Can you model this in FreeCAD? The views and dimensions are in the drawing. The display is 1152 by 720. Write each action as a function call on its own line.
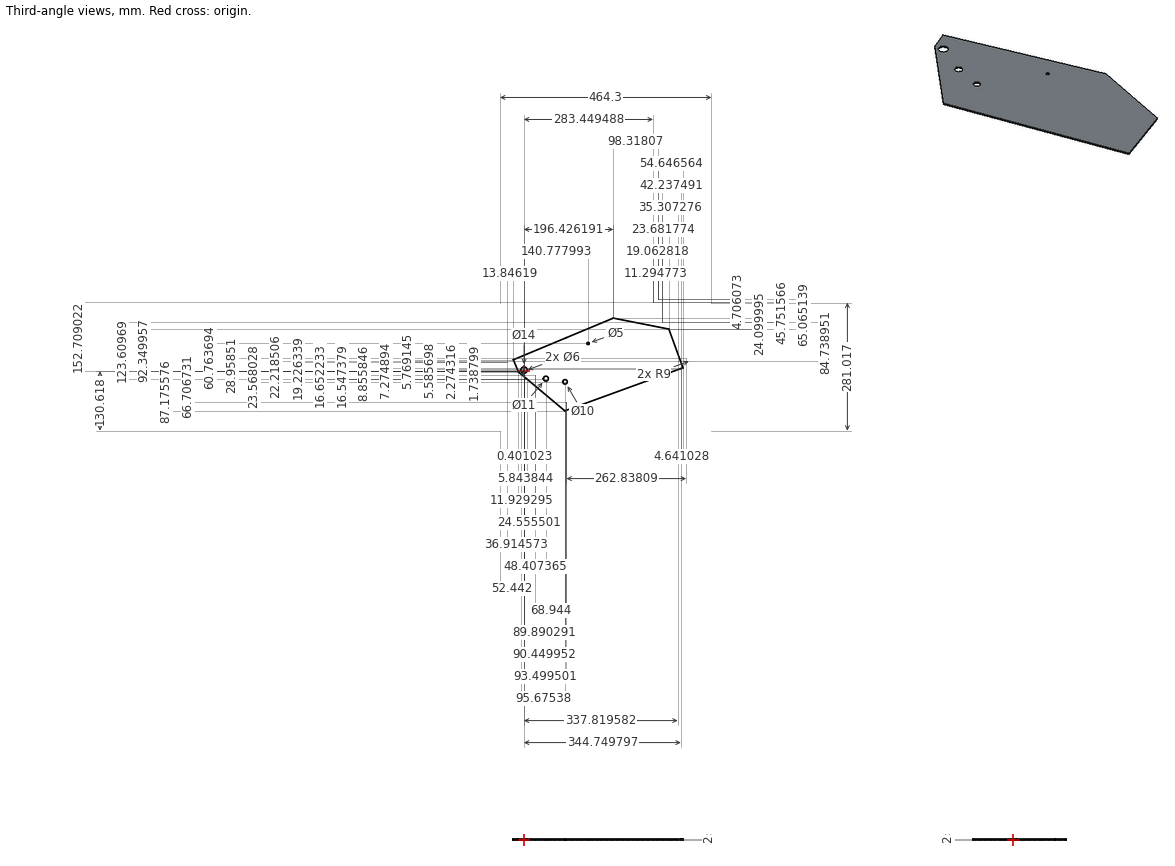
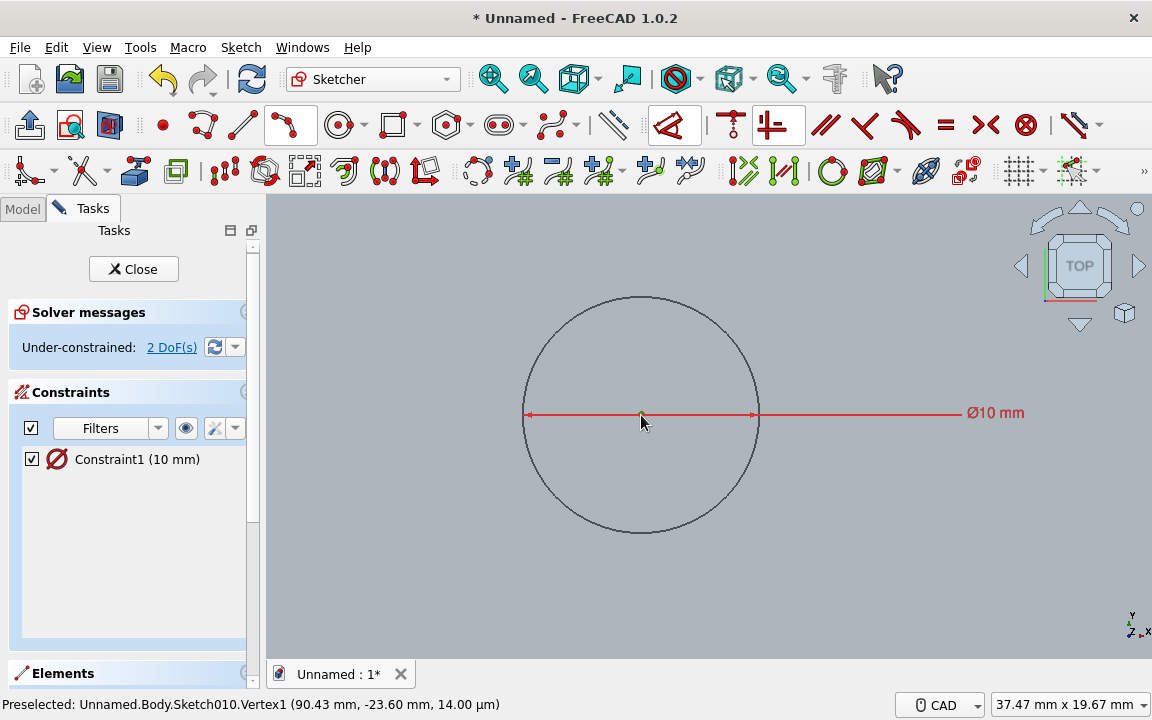
key(l)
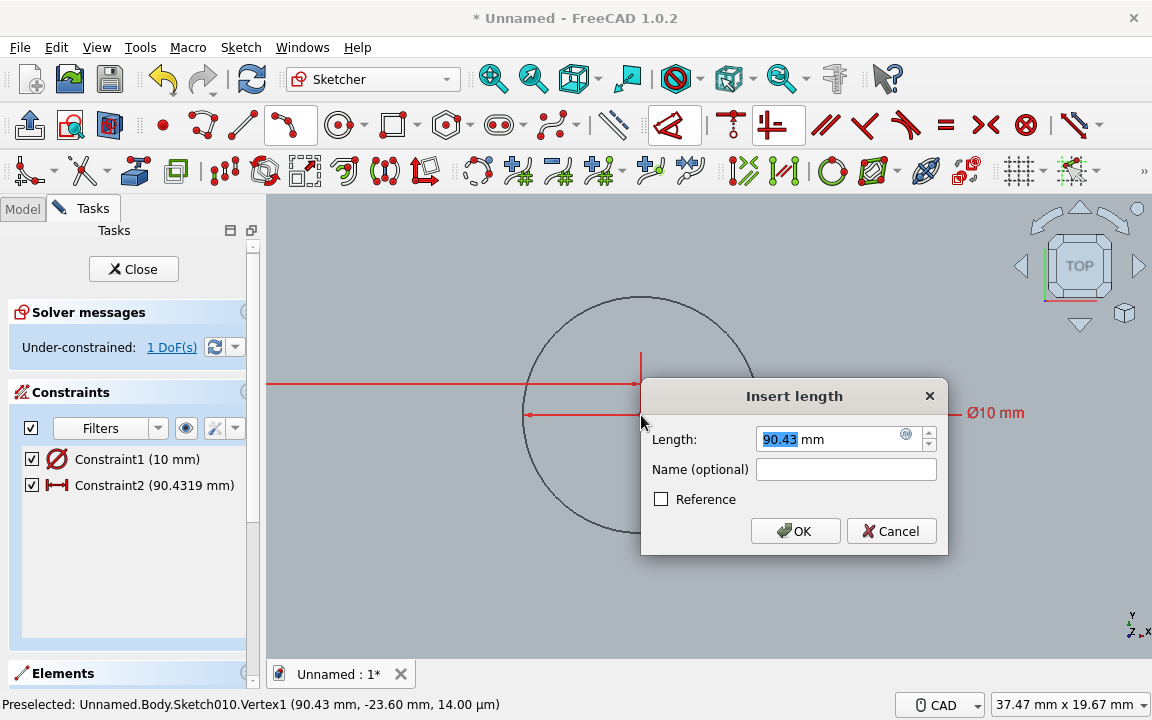
text(90.449952)
key(Return)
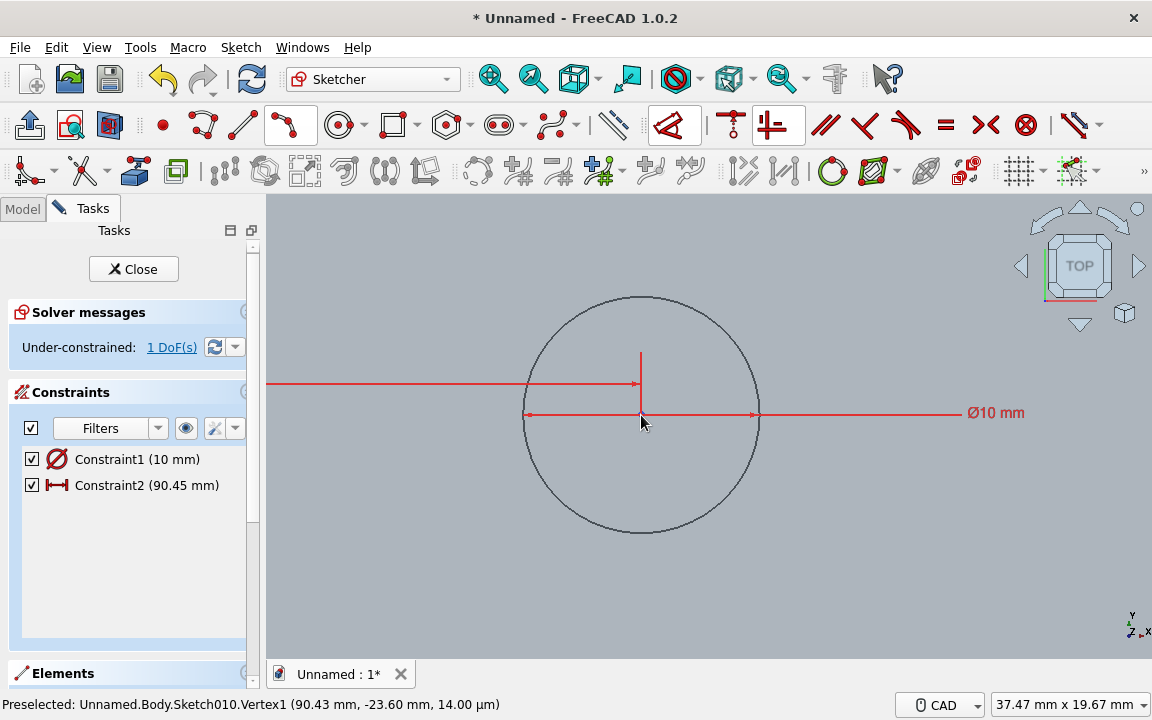
click(641, 415)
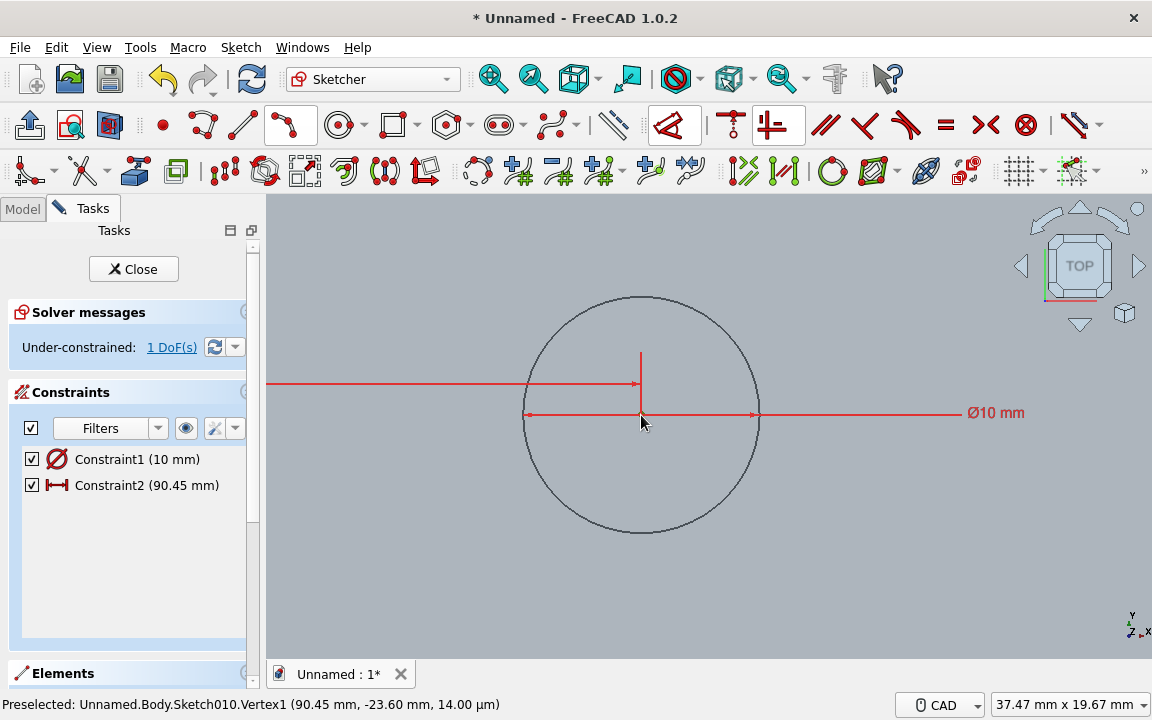
key(i)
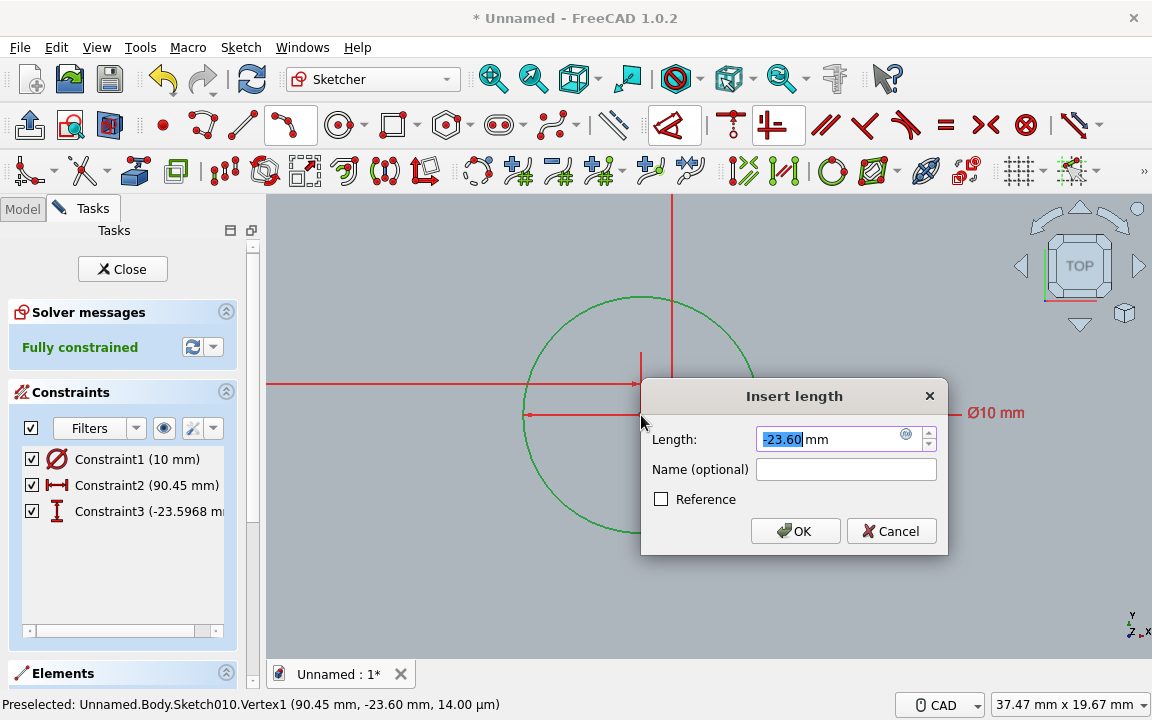
text(-23.568028)
key(Return)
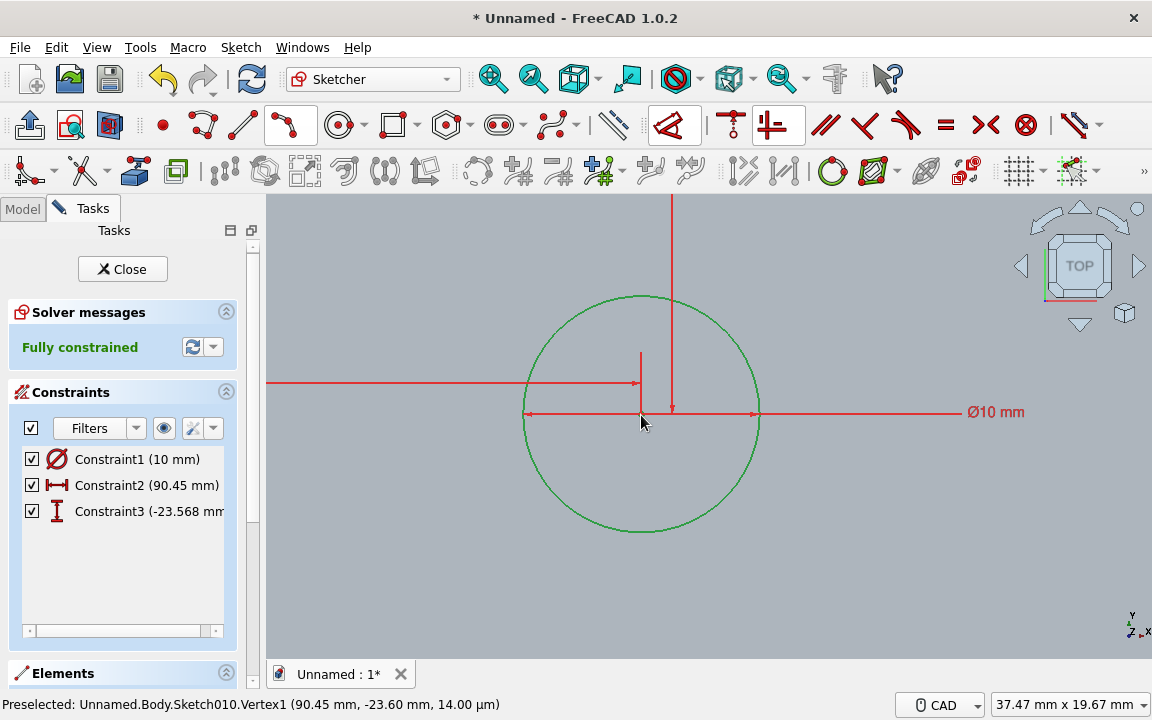
click(123, 269)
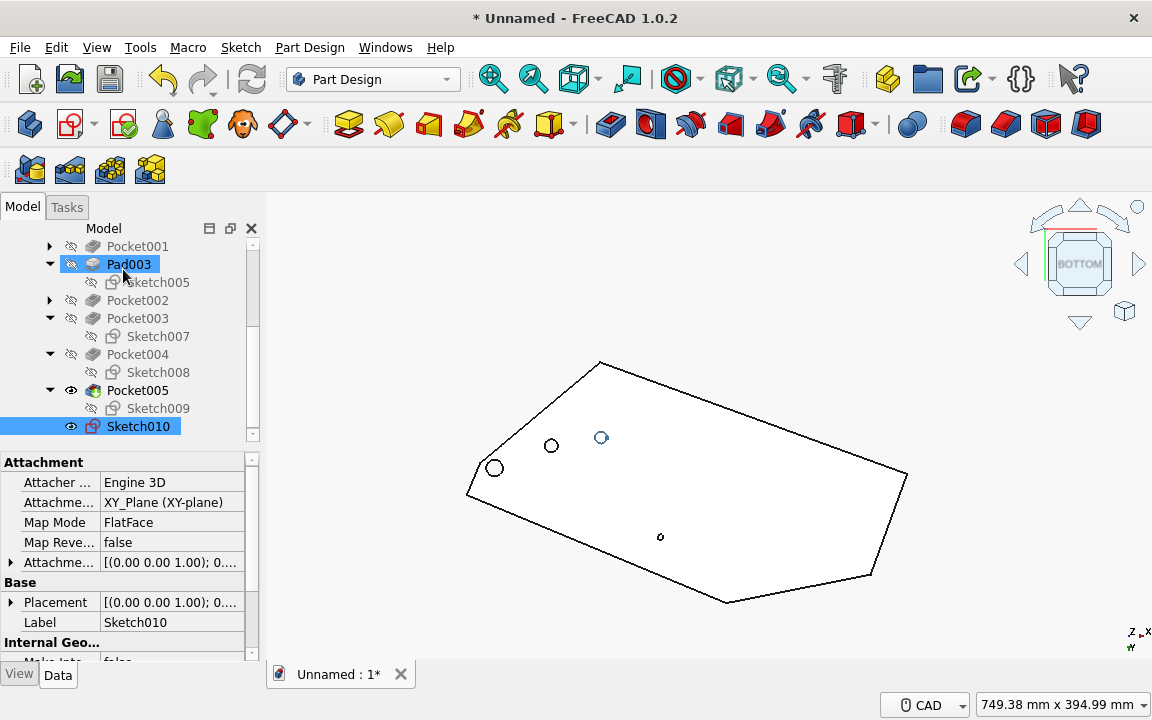
click(612, 124)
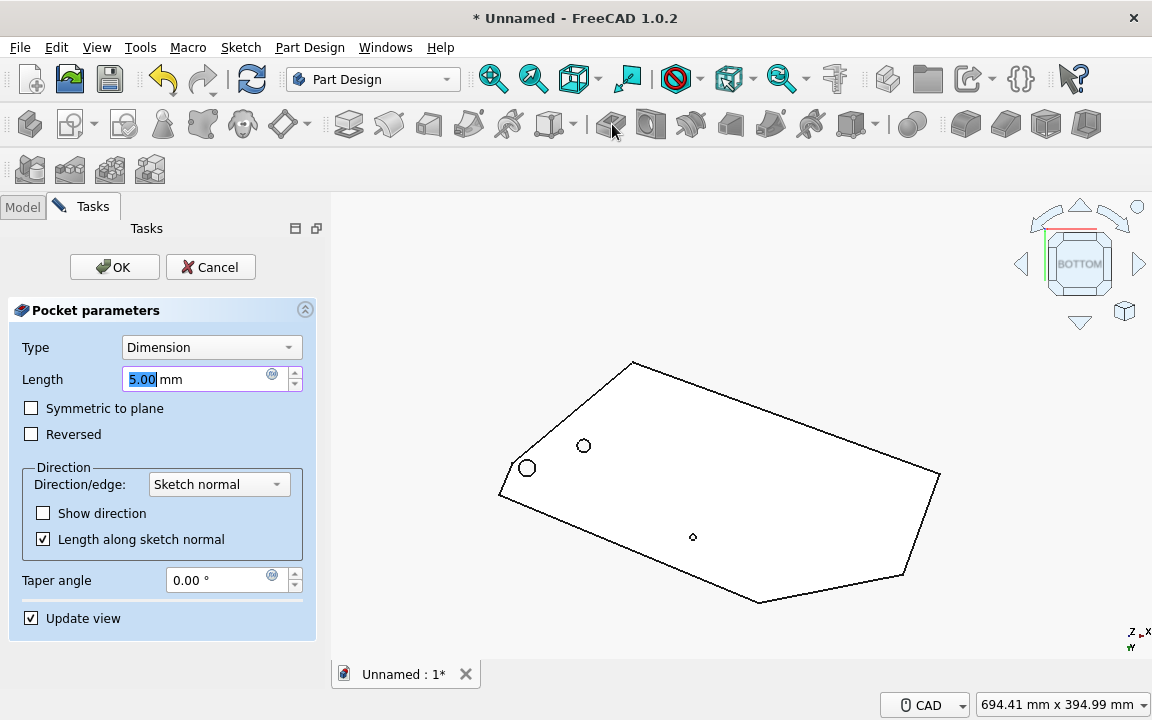
click(212, 348)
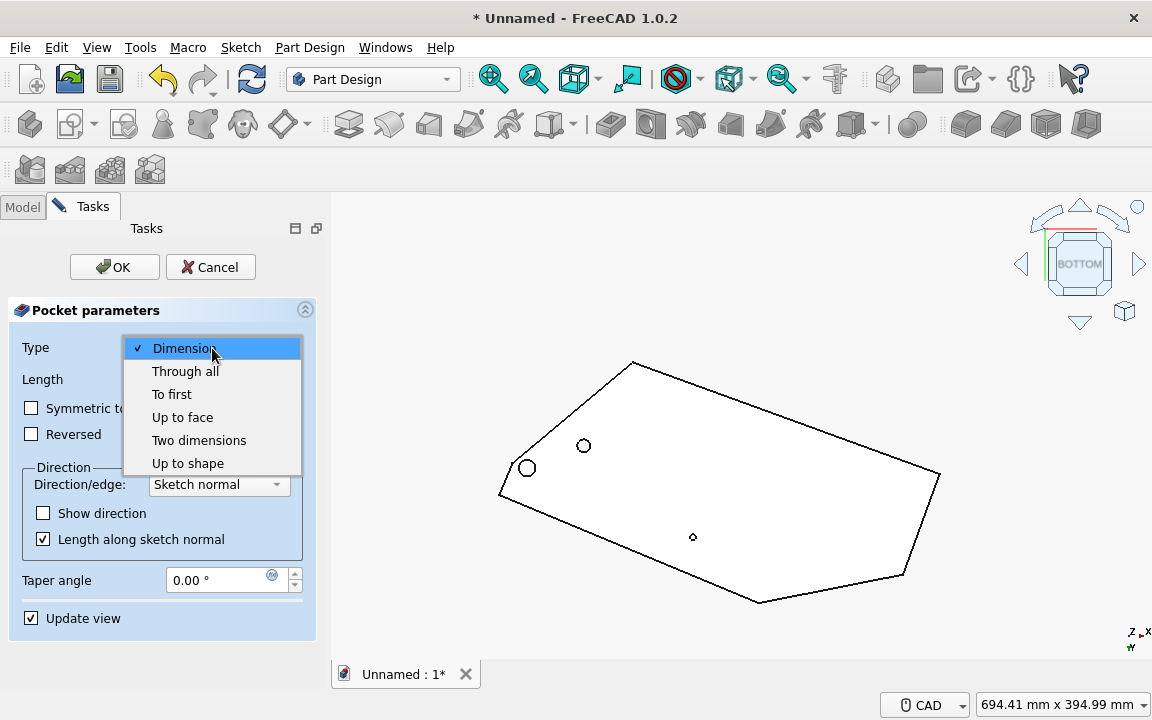
click(212, 372)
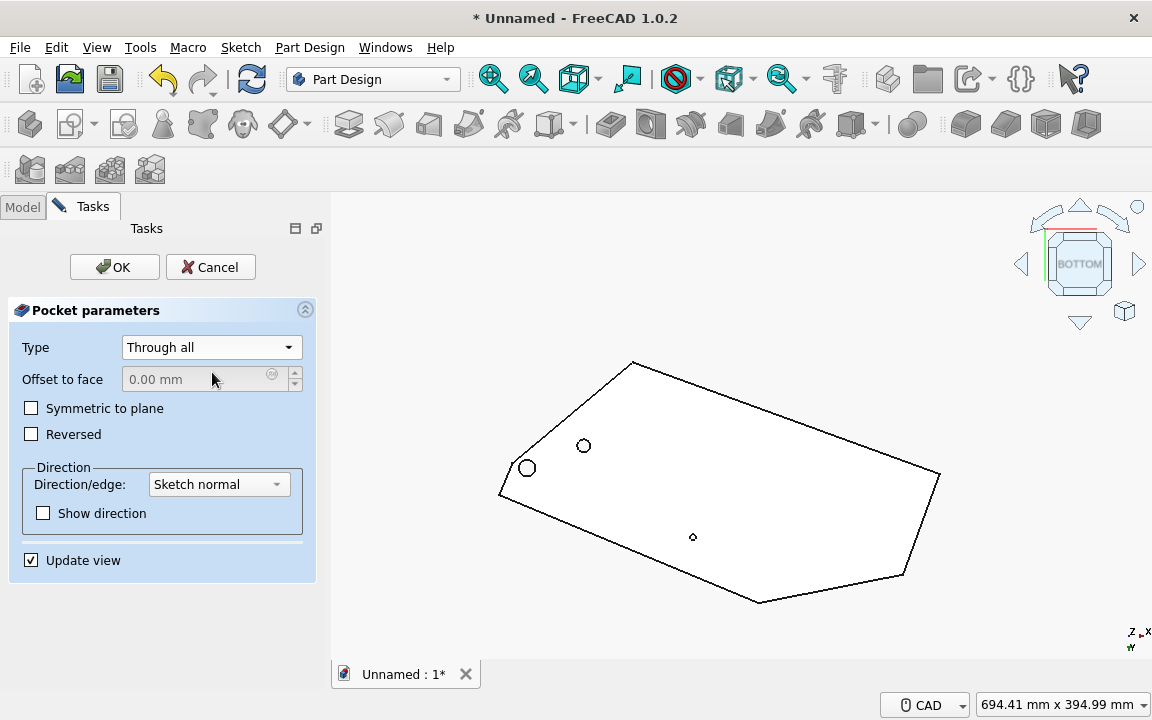
click(30, 434)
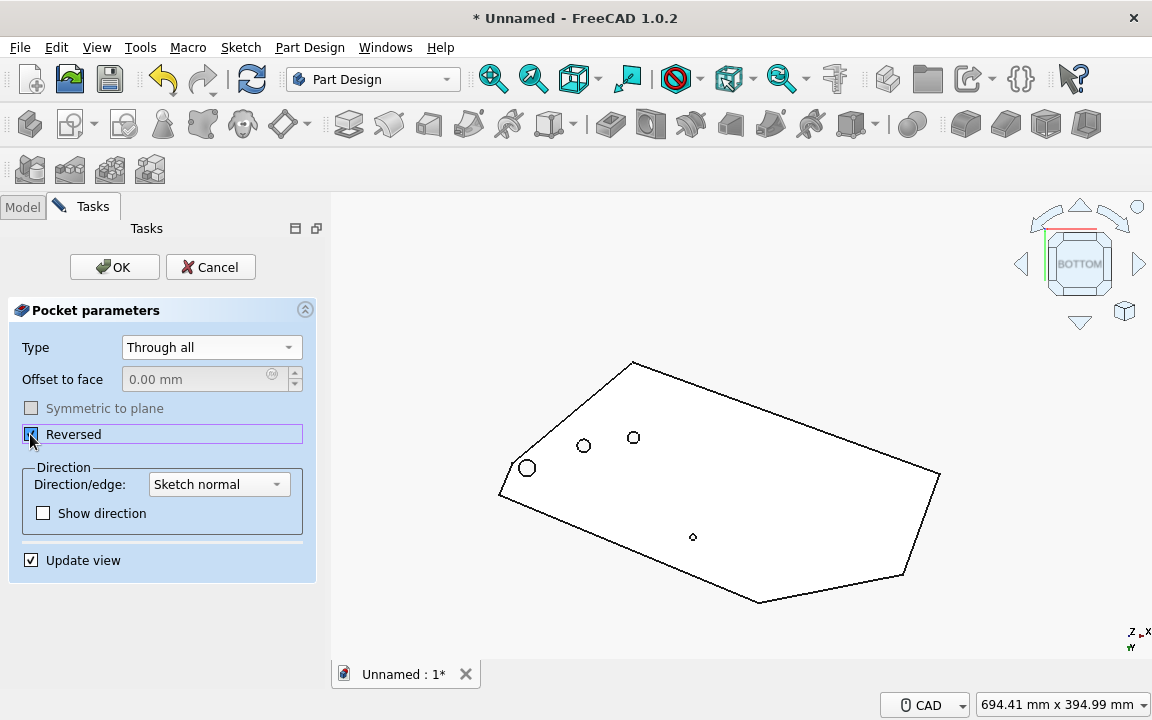
click(115, 267)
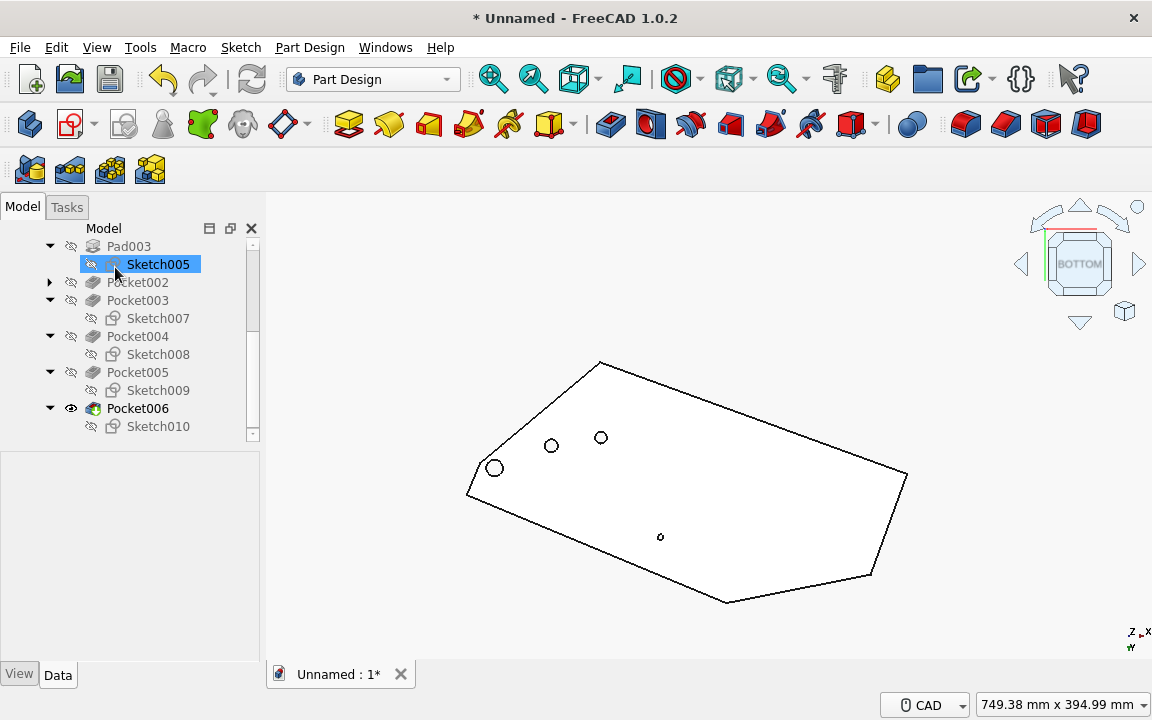
key(0)